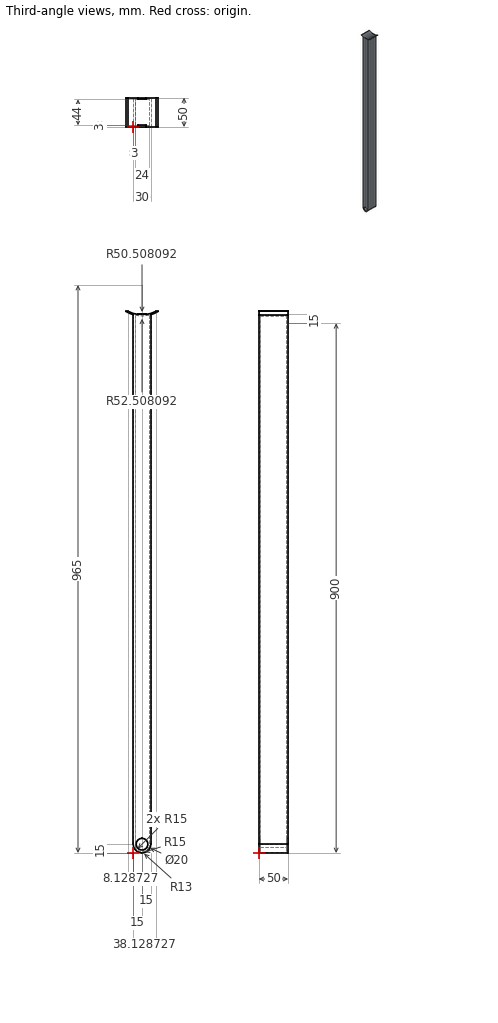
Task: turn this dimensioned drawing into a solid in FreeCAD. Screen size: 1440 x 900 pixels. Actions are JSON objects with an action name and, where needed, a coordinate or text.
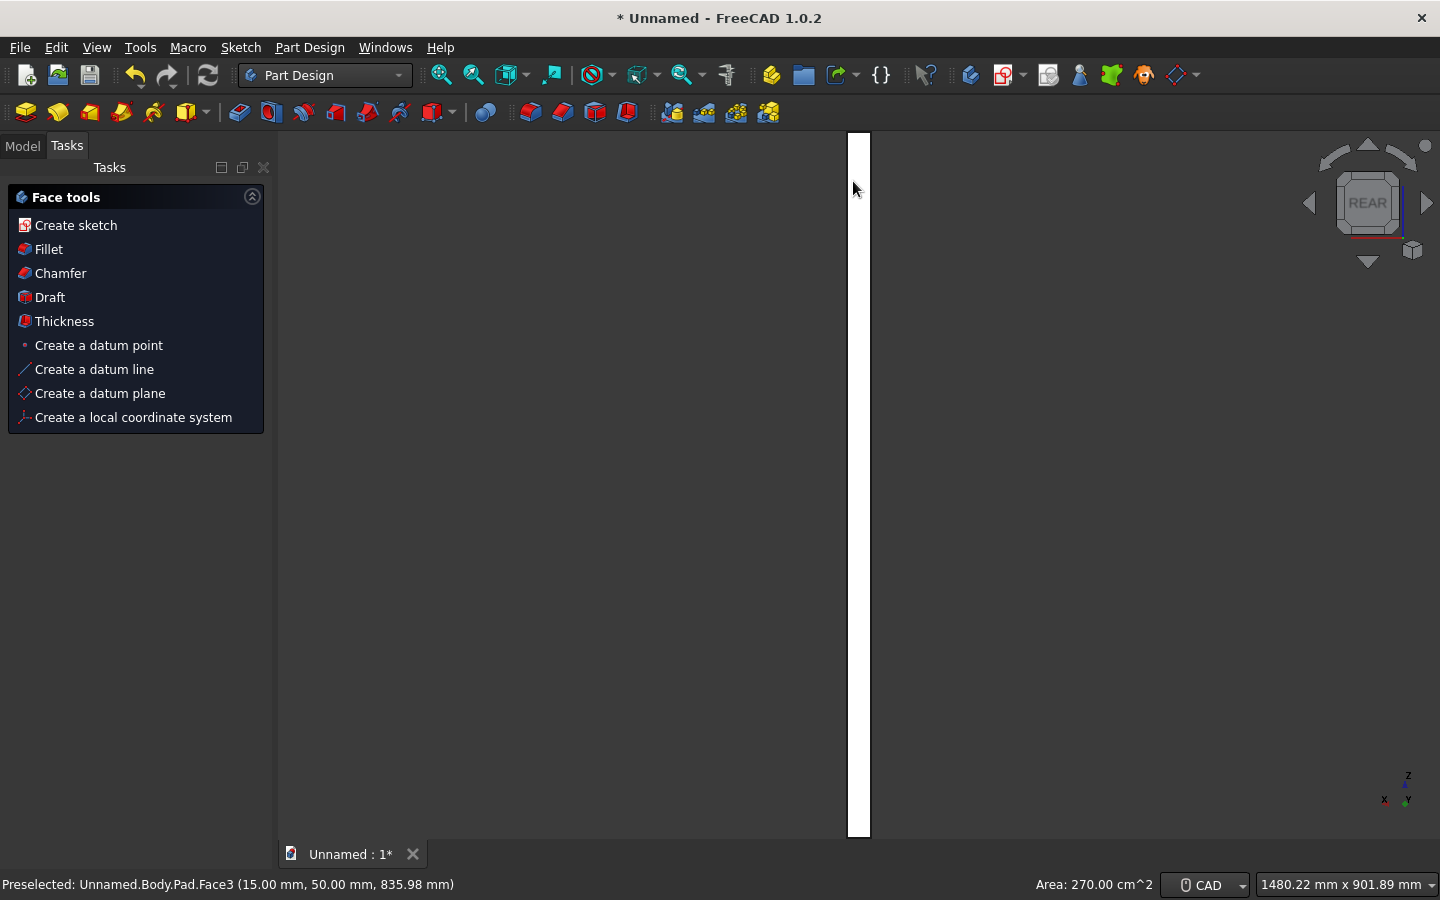
{"action": "left_click", "coordinate": [1004, 76]}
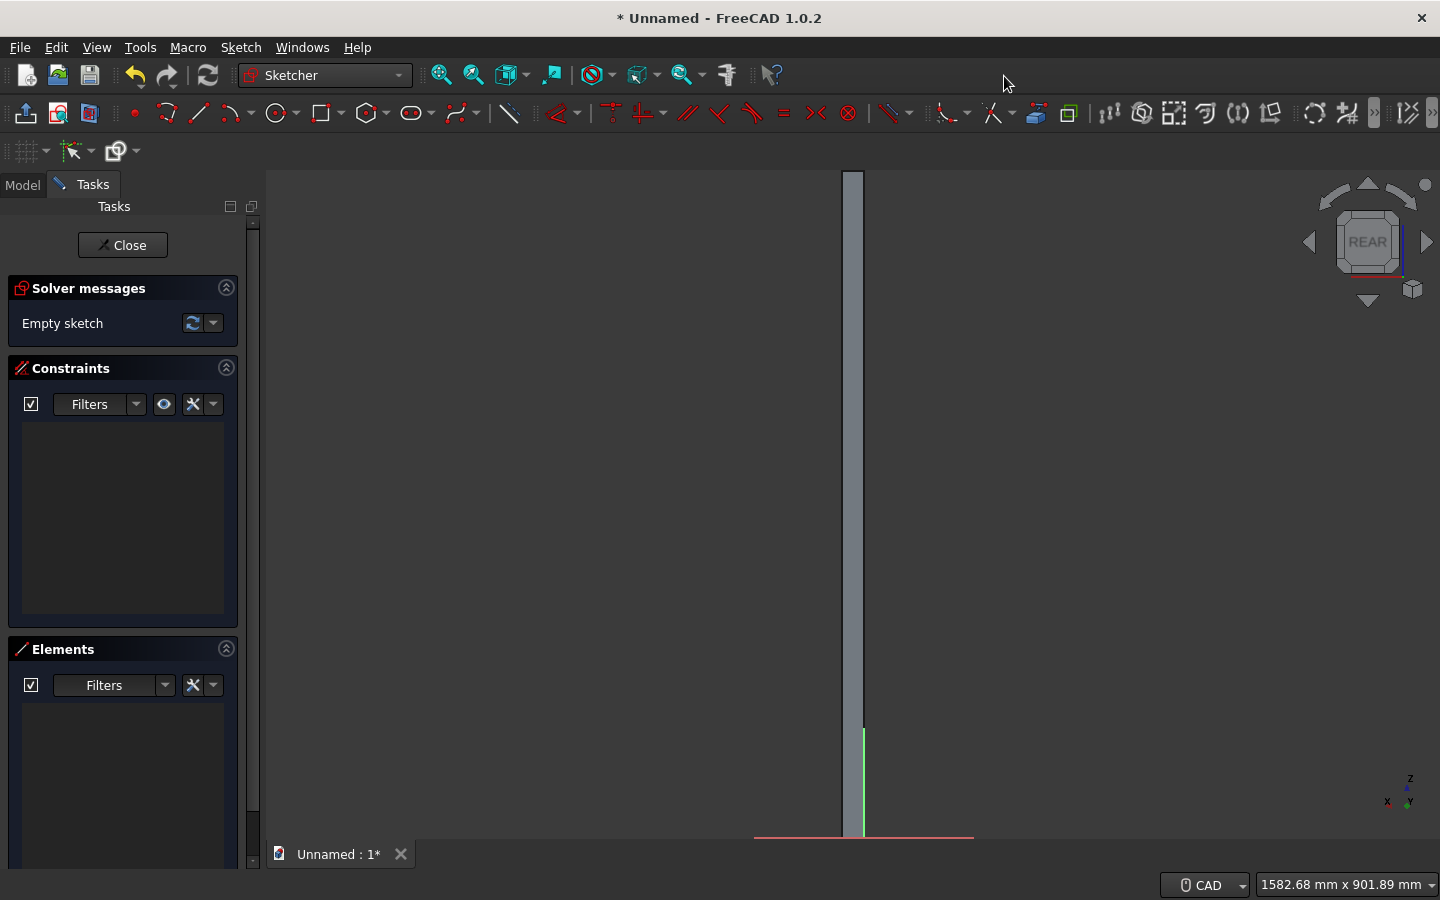
{"action": "scroll", "coordinate": [784, 504], "scroll_direction": "down", "scroll_amount": 5}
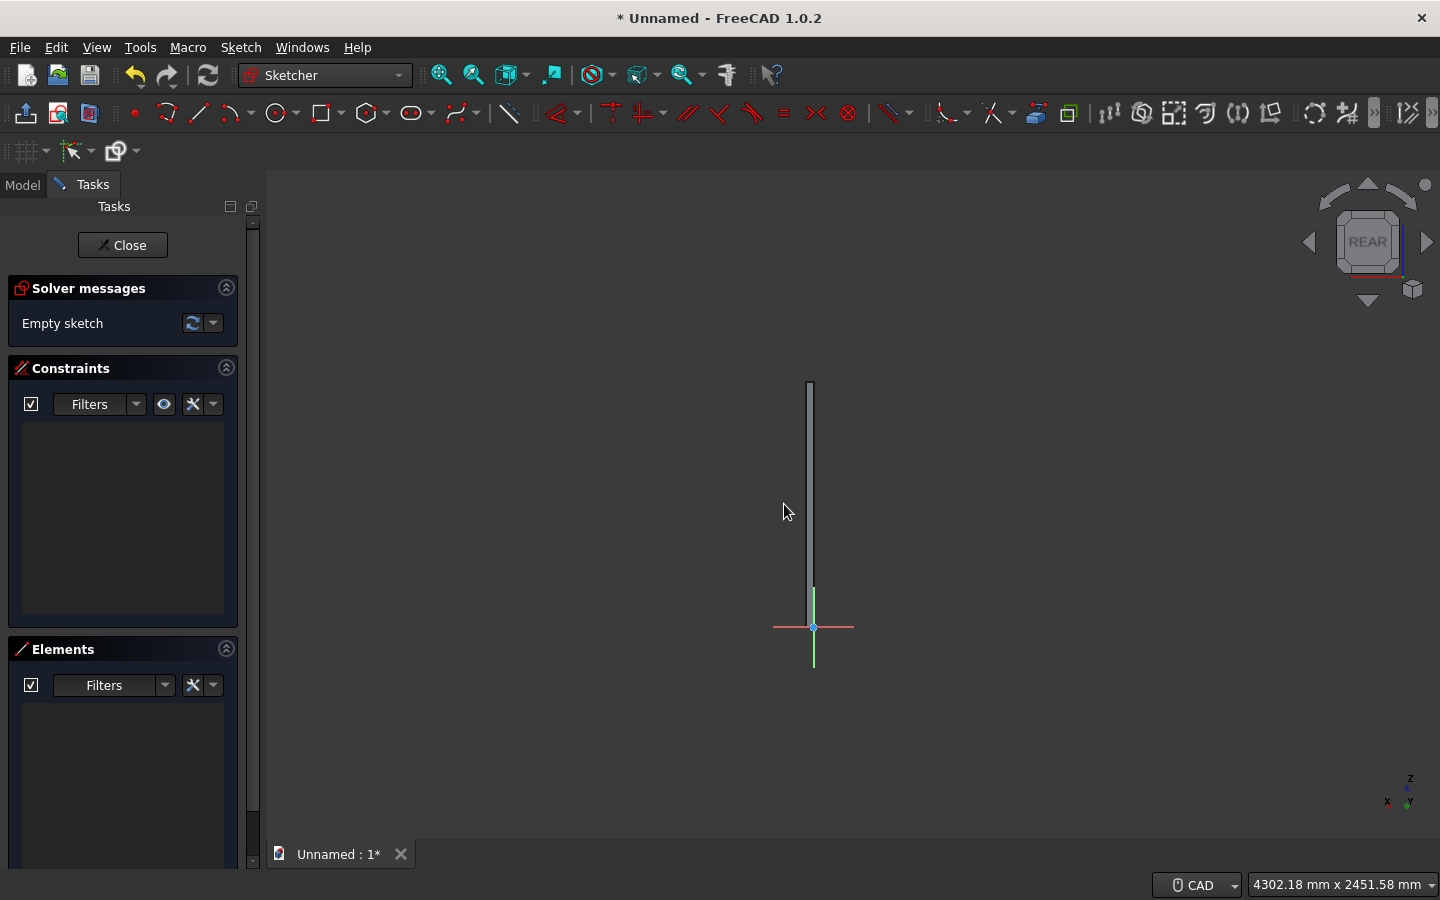
{"action": "scroll", "coordinate": [811, 630], "scroll_direction": "up", "scroll_amount": 15}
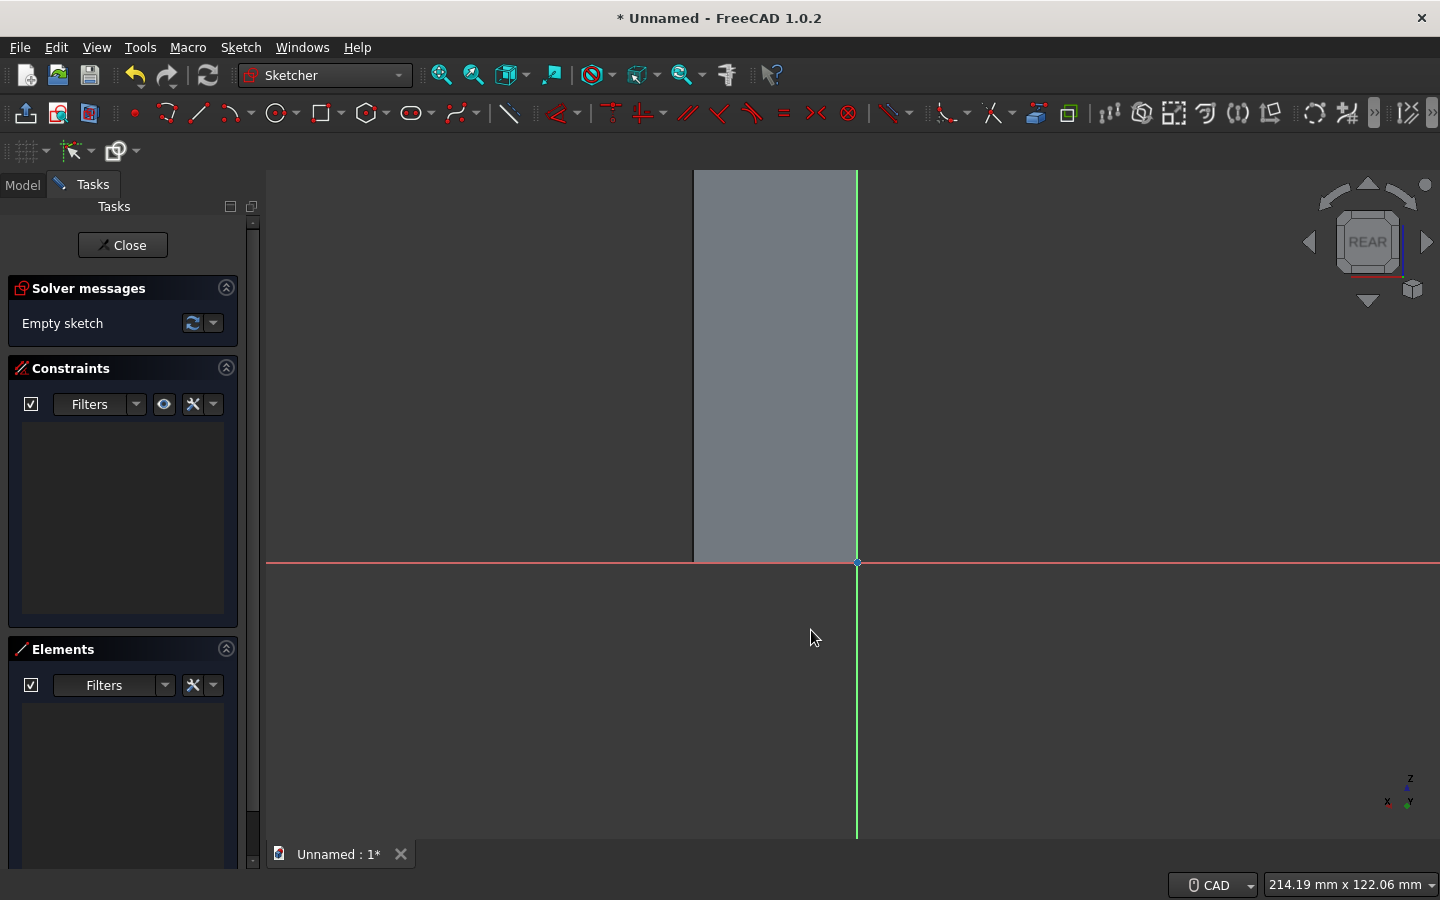
{"action": "scroll", "coordinate": [771, 490], "scroll_direction": "up", "scroll_amount": 6}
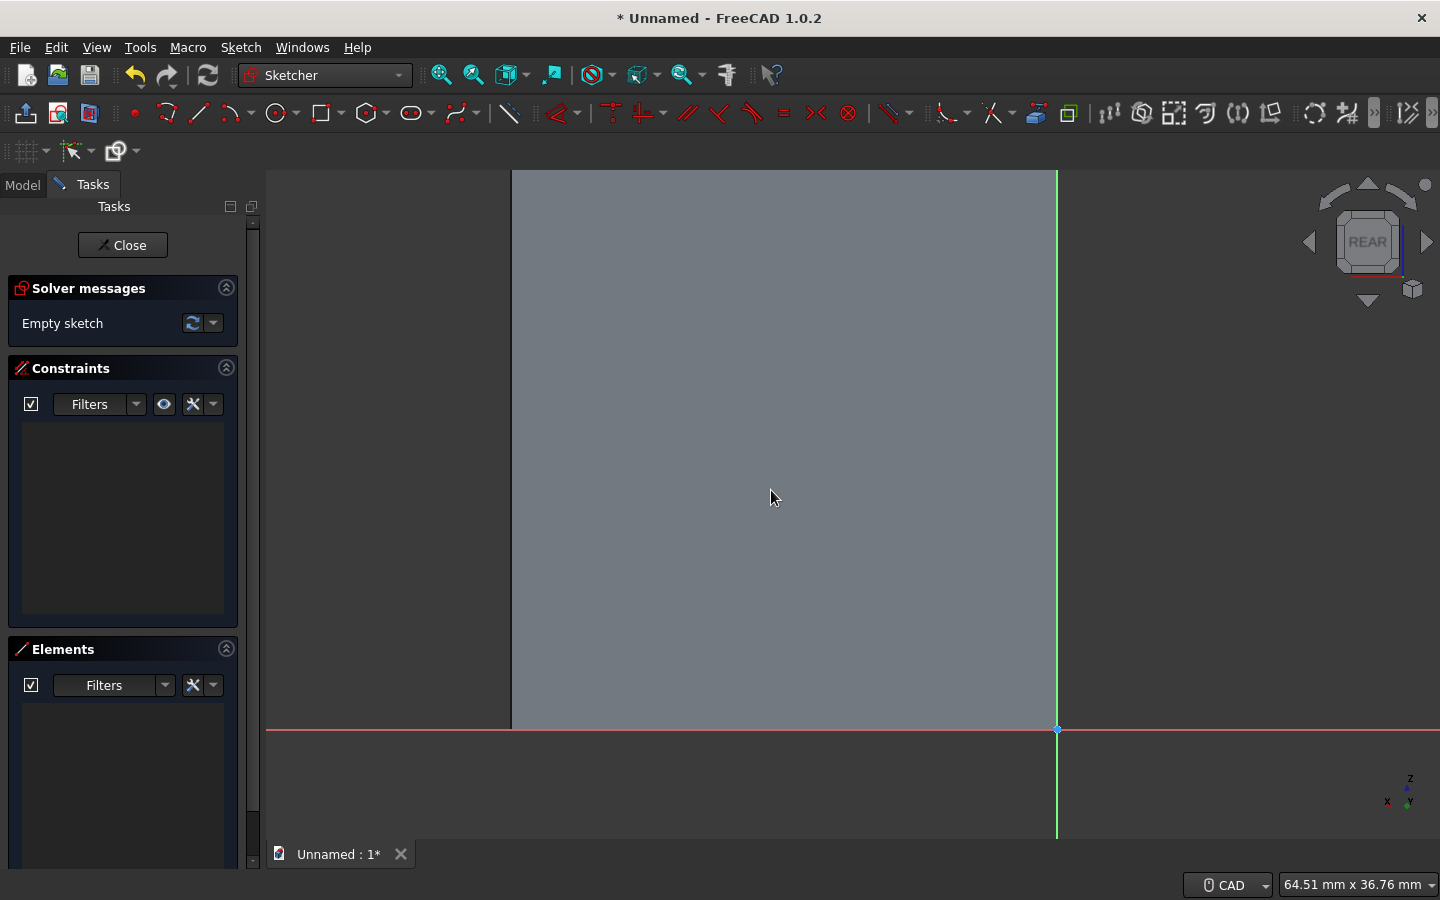
{"action": "left_click", "coordinate": [168, 114]}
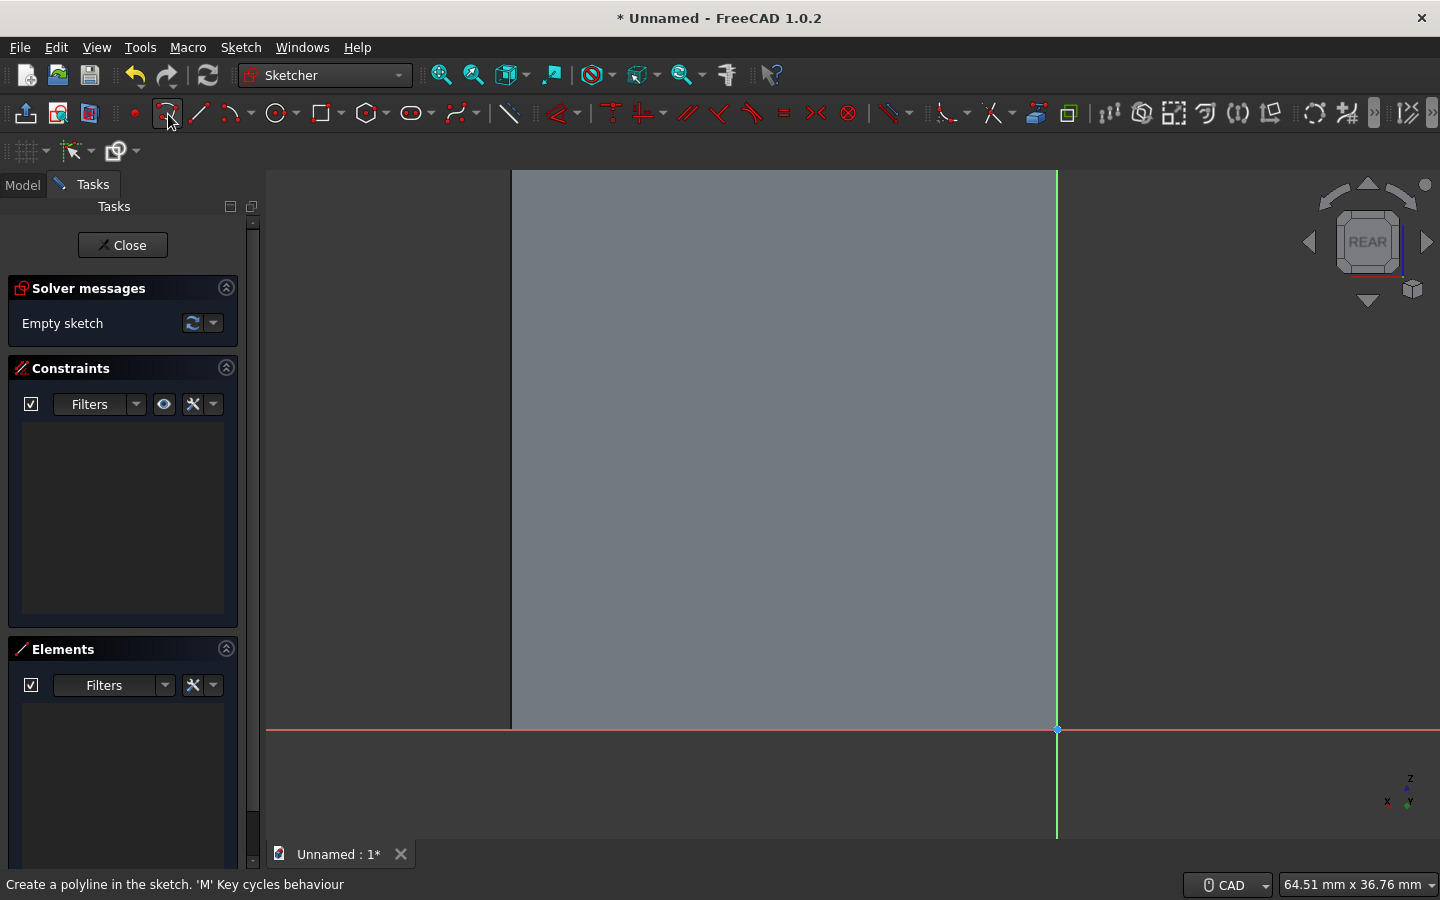
{"action": "left_click", "coordinate": [784, 730]}
{"action": "left_click", "coordinate": [1057, 730]}
{"action": "left_click", "coordinate": [1048, 457]}
{"action": "right_click", "coordinate": [1048, 457]}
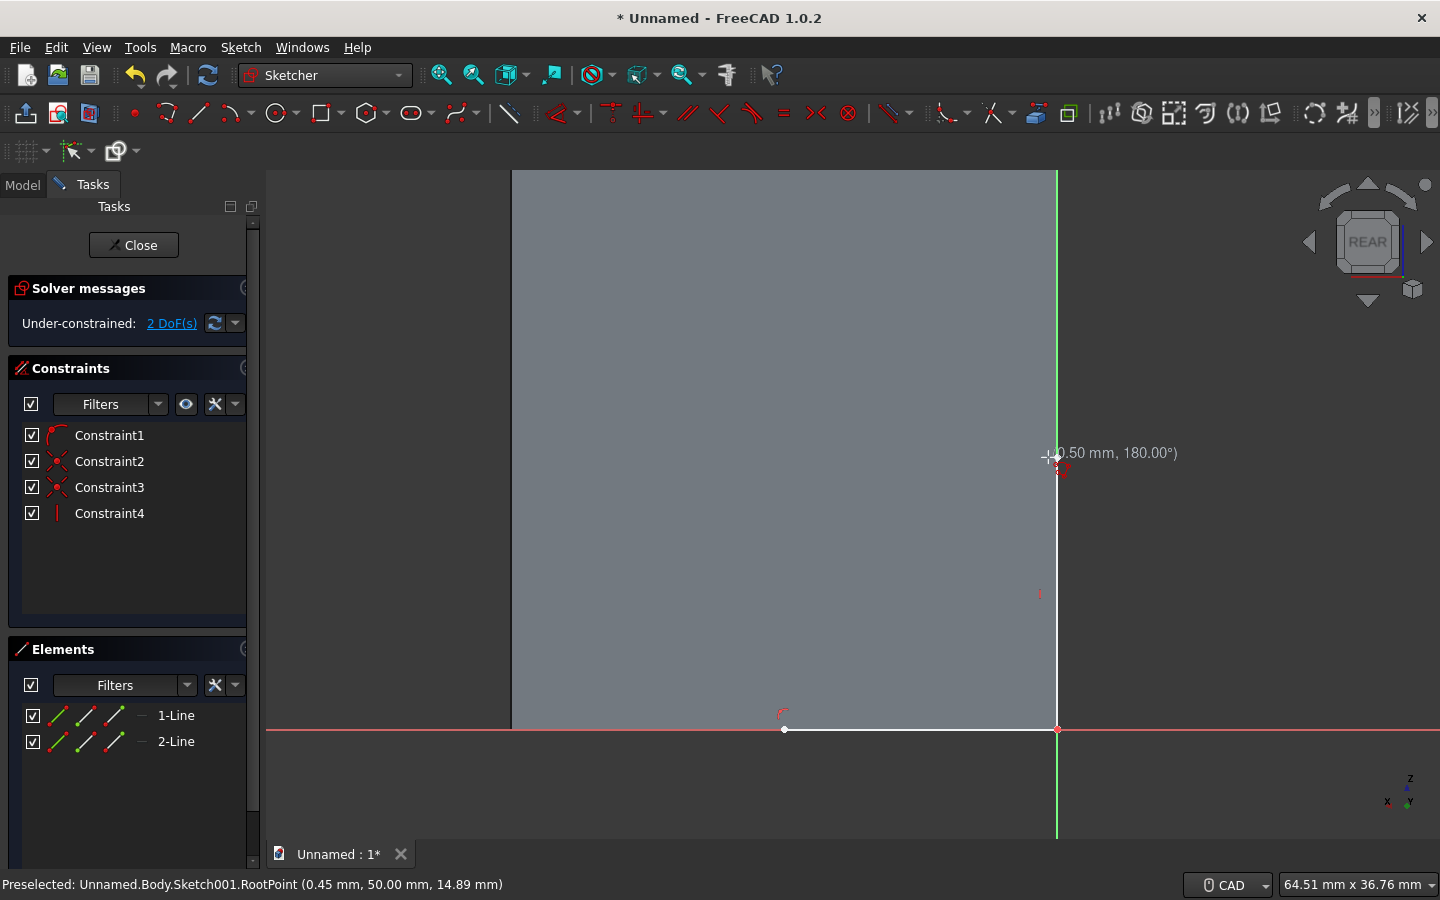
{"action": "left_click", "coordinate": [254, 114]}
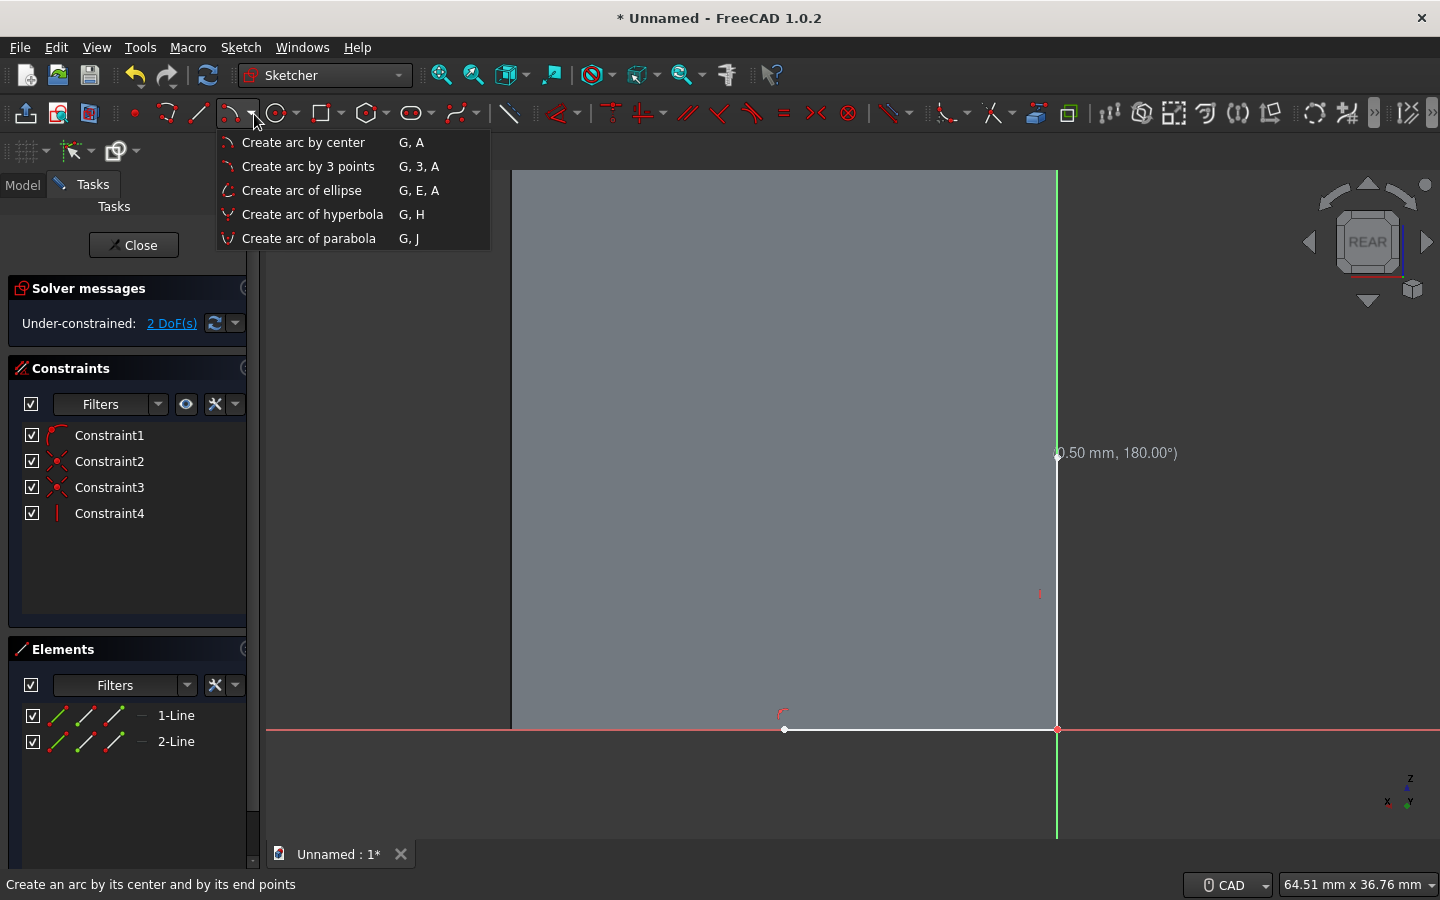
{"action": "left_click", "coordinate": [354, 166]}